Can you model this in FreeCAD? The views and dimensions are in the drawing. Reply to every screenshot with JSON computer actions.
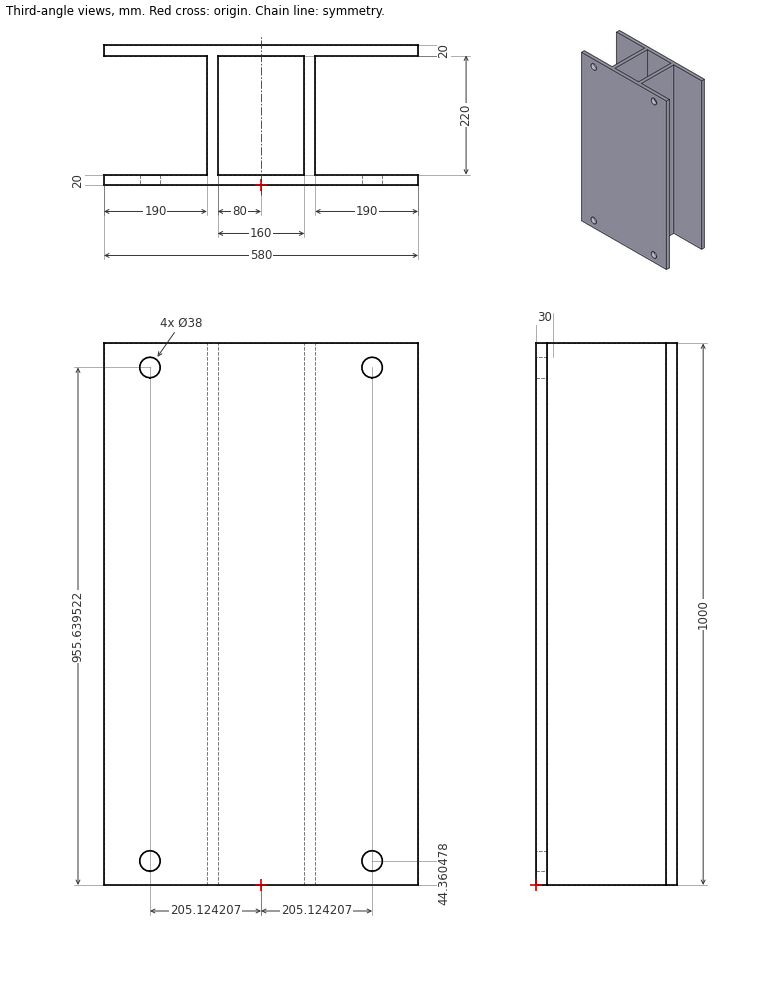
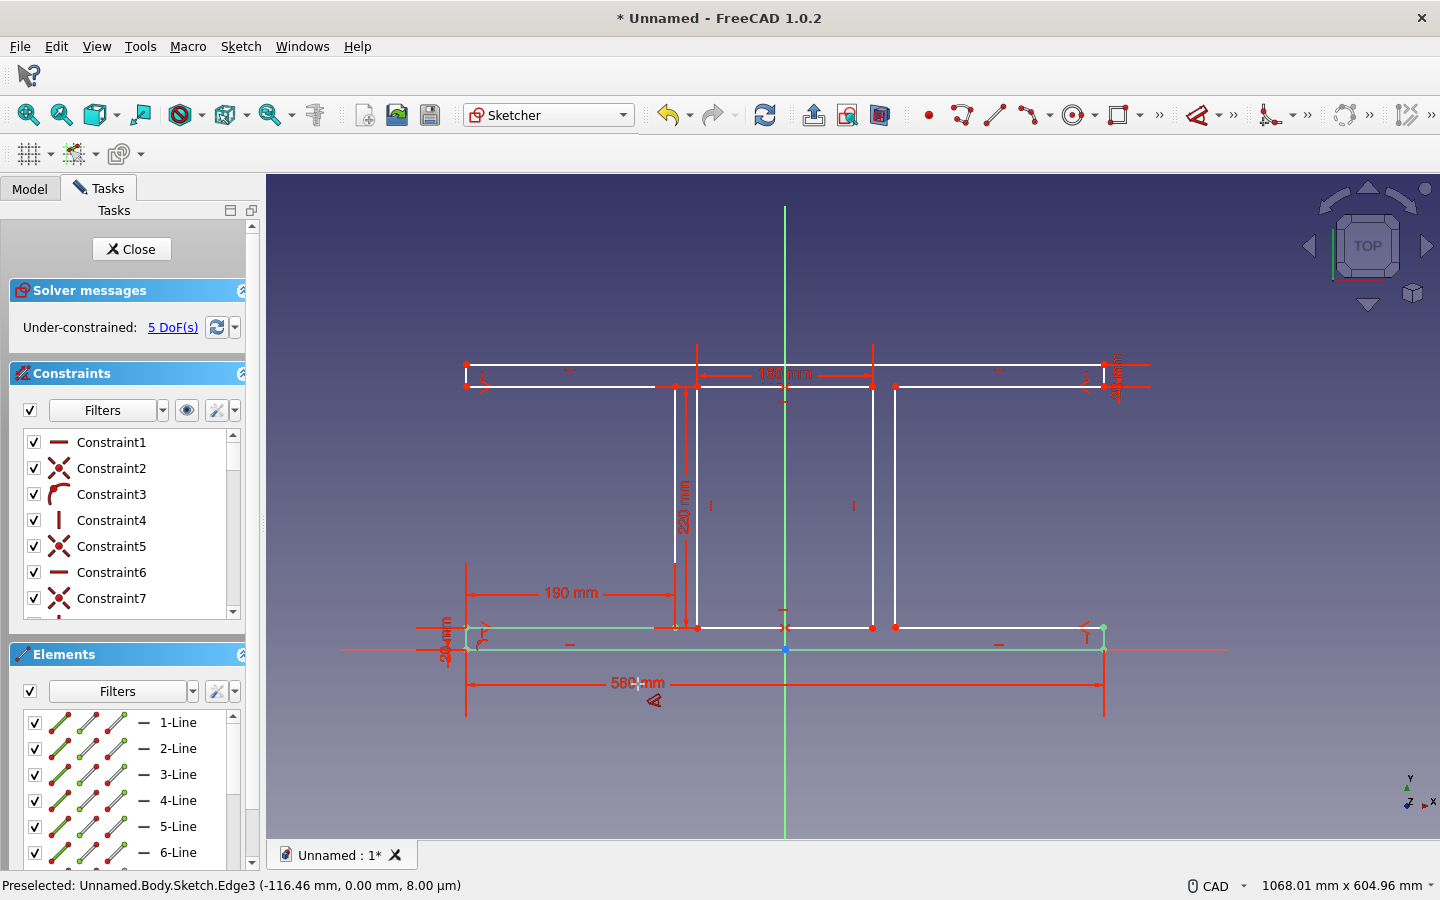
{"action": "left_click", "coordinate": [1041, 628]}
{"action": "left_click", "coordinate": [999, 594]}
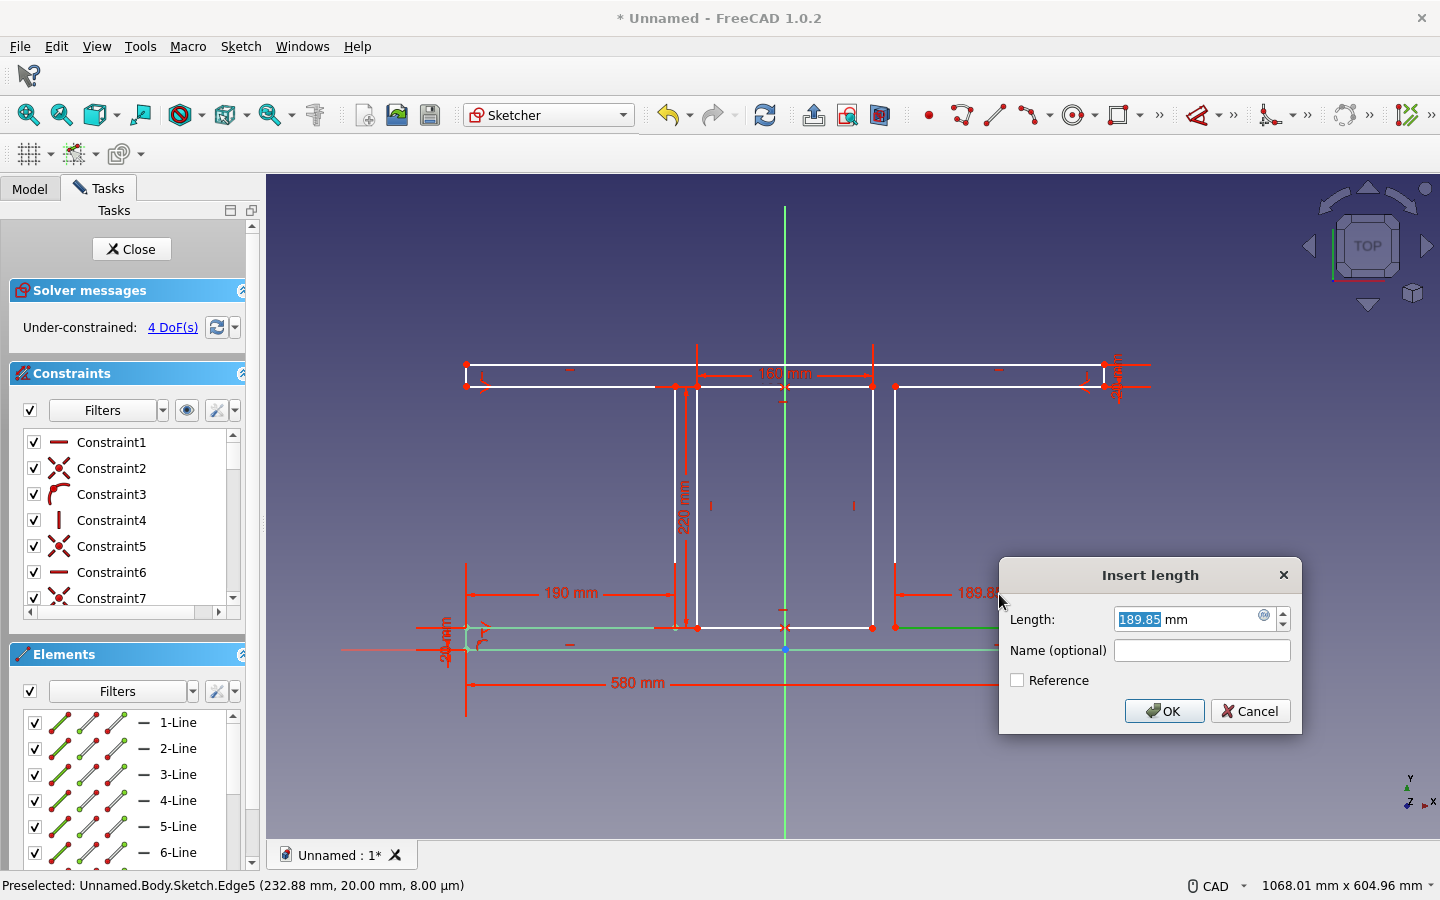
{"action": "type", "text": "190"}
{"action": "key", "text": "Return"}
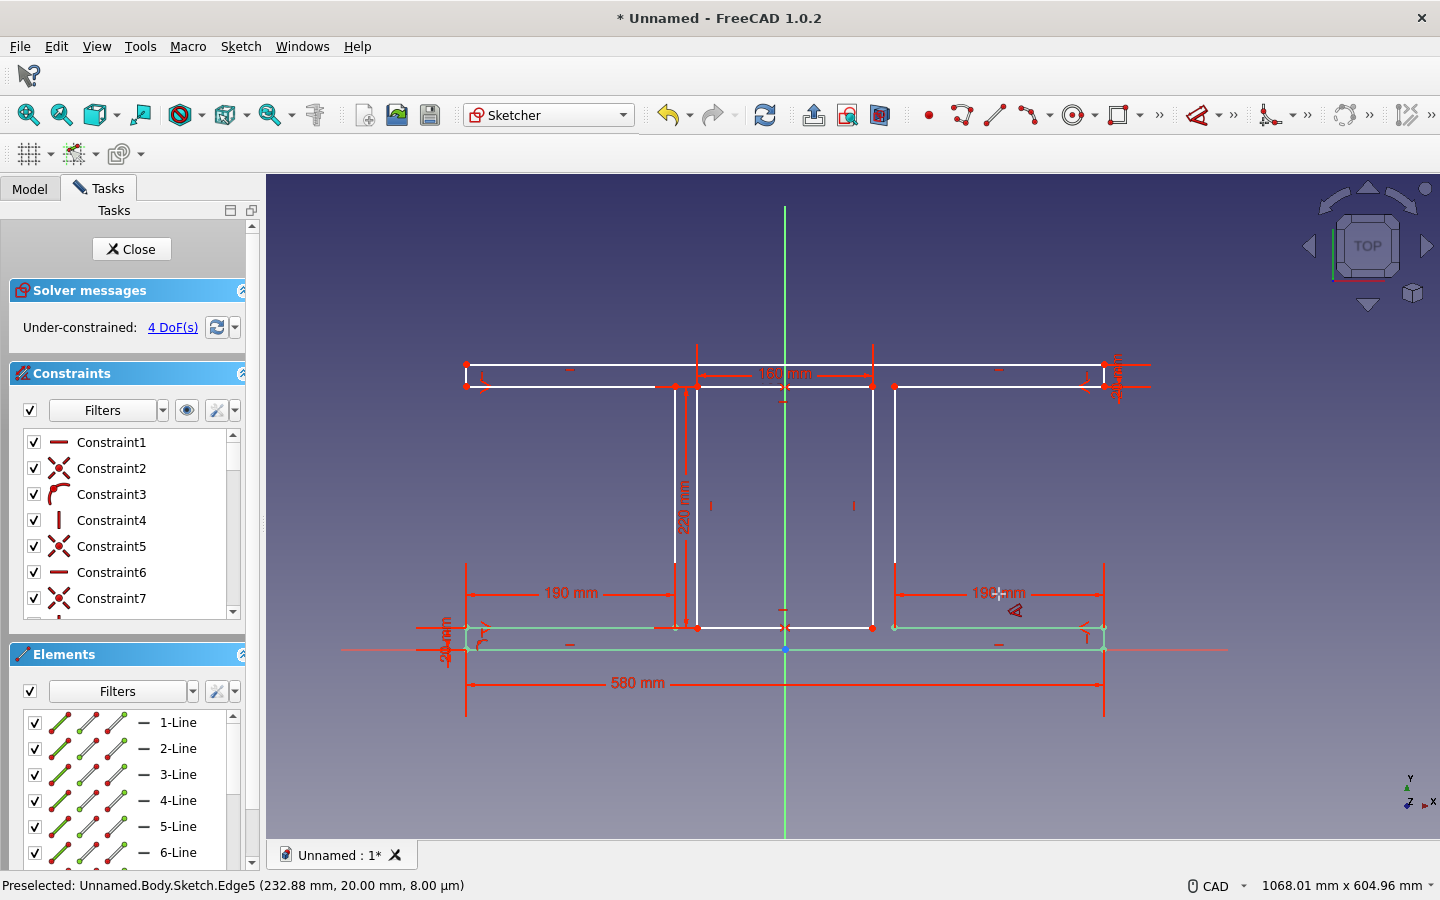
{"action": "left_click", "coordinate": [895, 555]}
{"action": "left_click", "coordinate": [929, 507]}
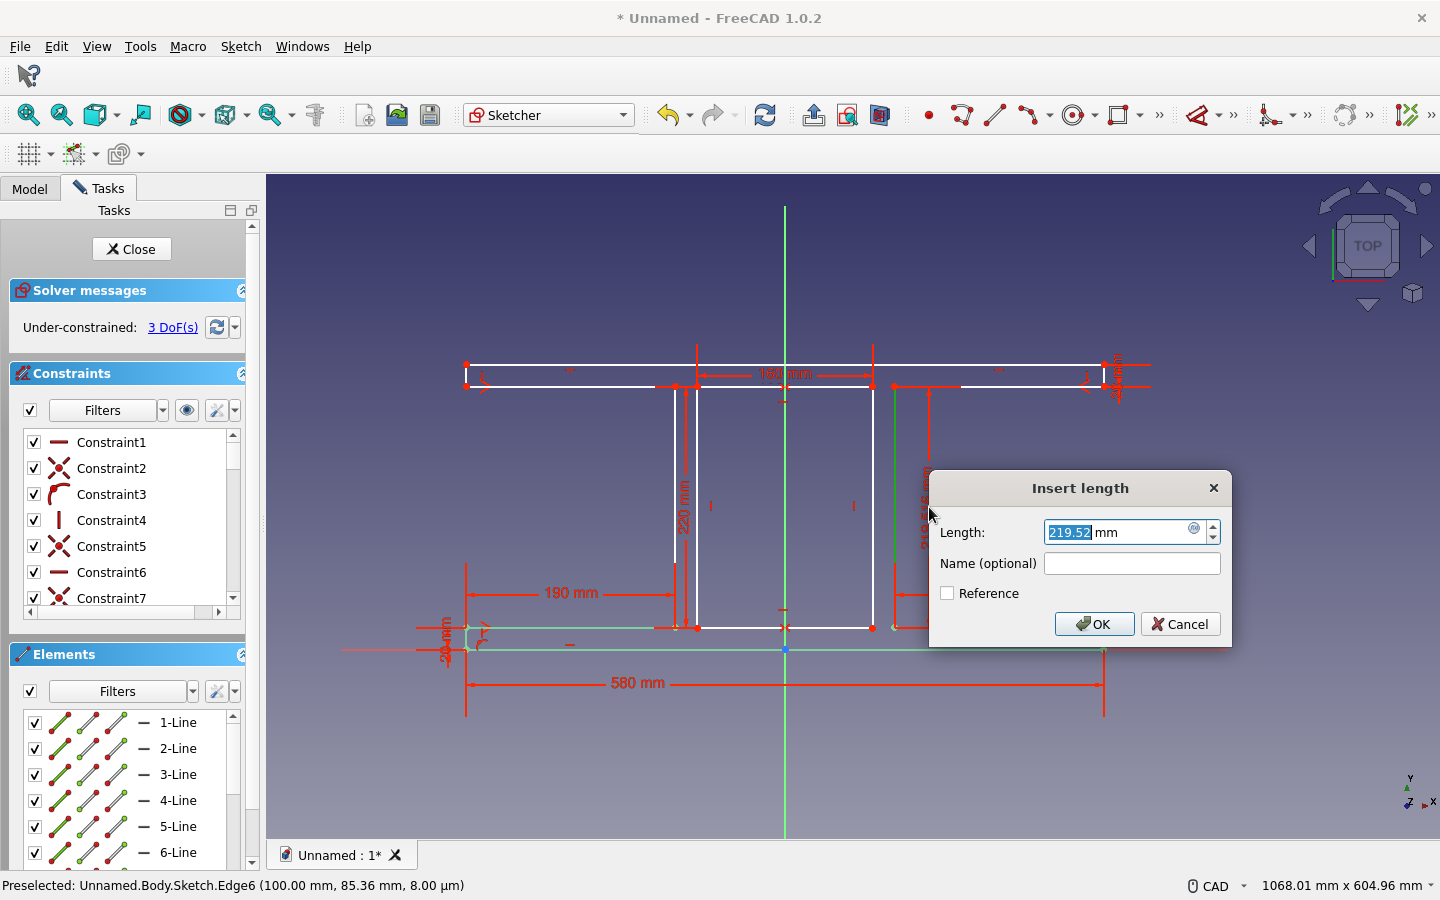
{"action": "type", "text": "220"}
{"action": "key", "text": "Return"}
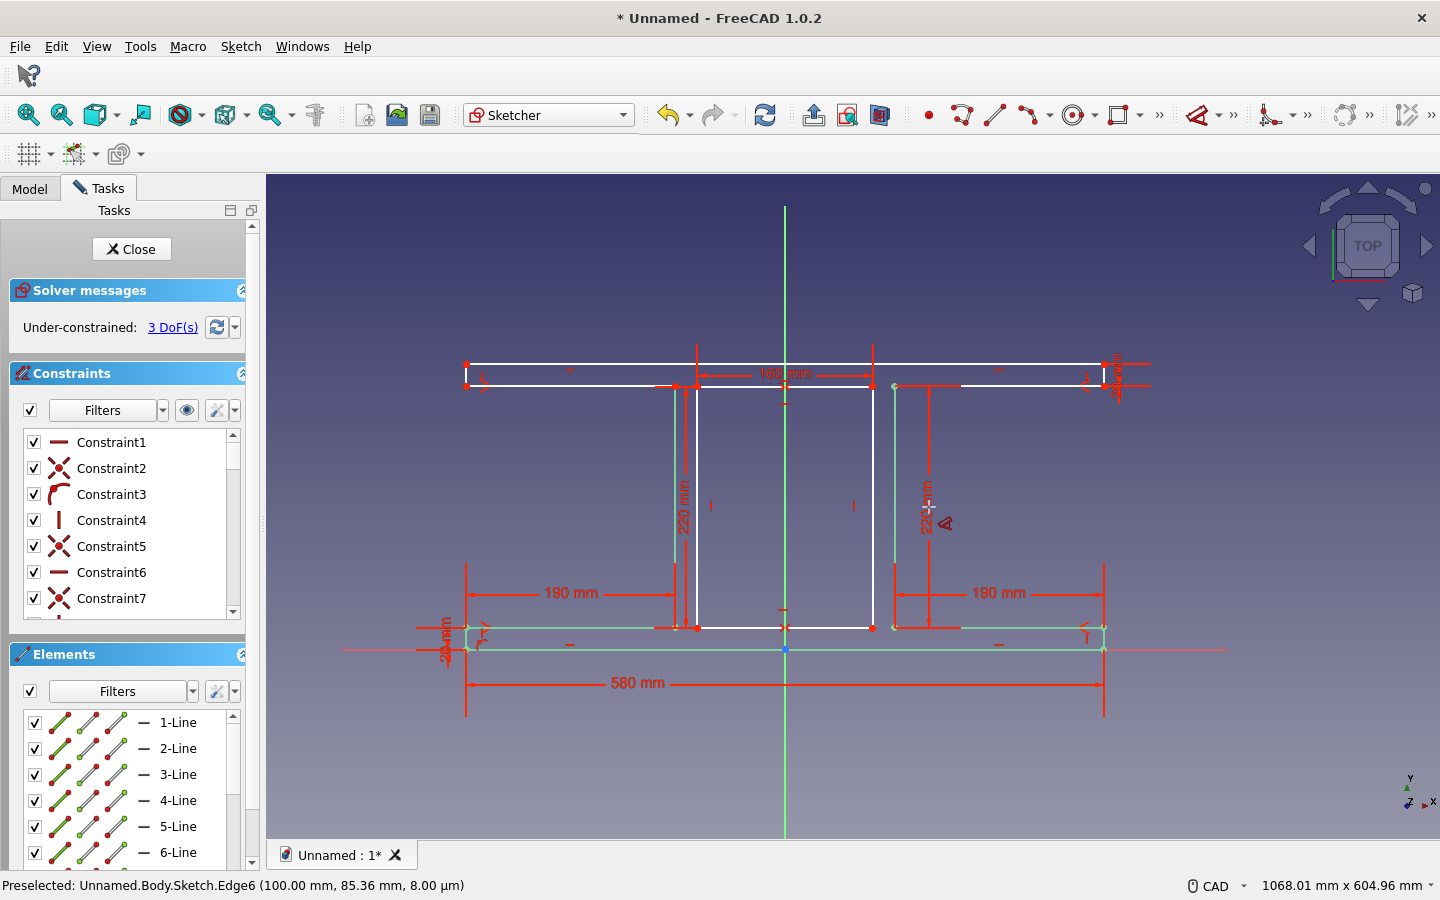
{"action": "left_click", "coordinate": [958, 386]}
{"action": "left_click", "coordinate": [999, 420]}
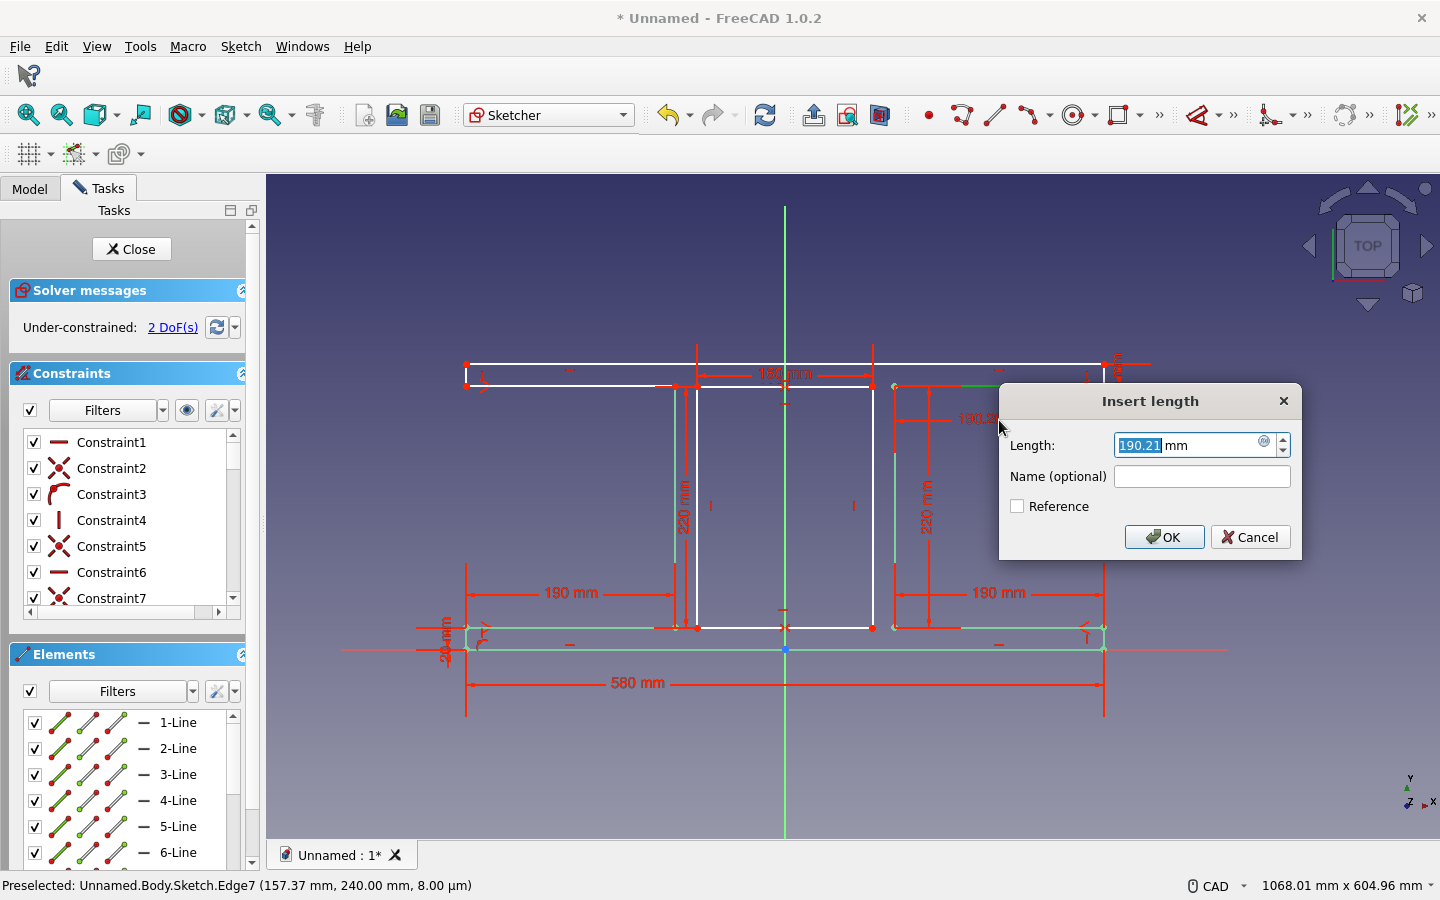
{"action": "type", "text": "190"}
{"action": "key", "text": "Return"}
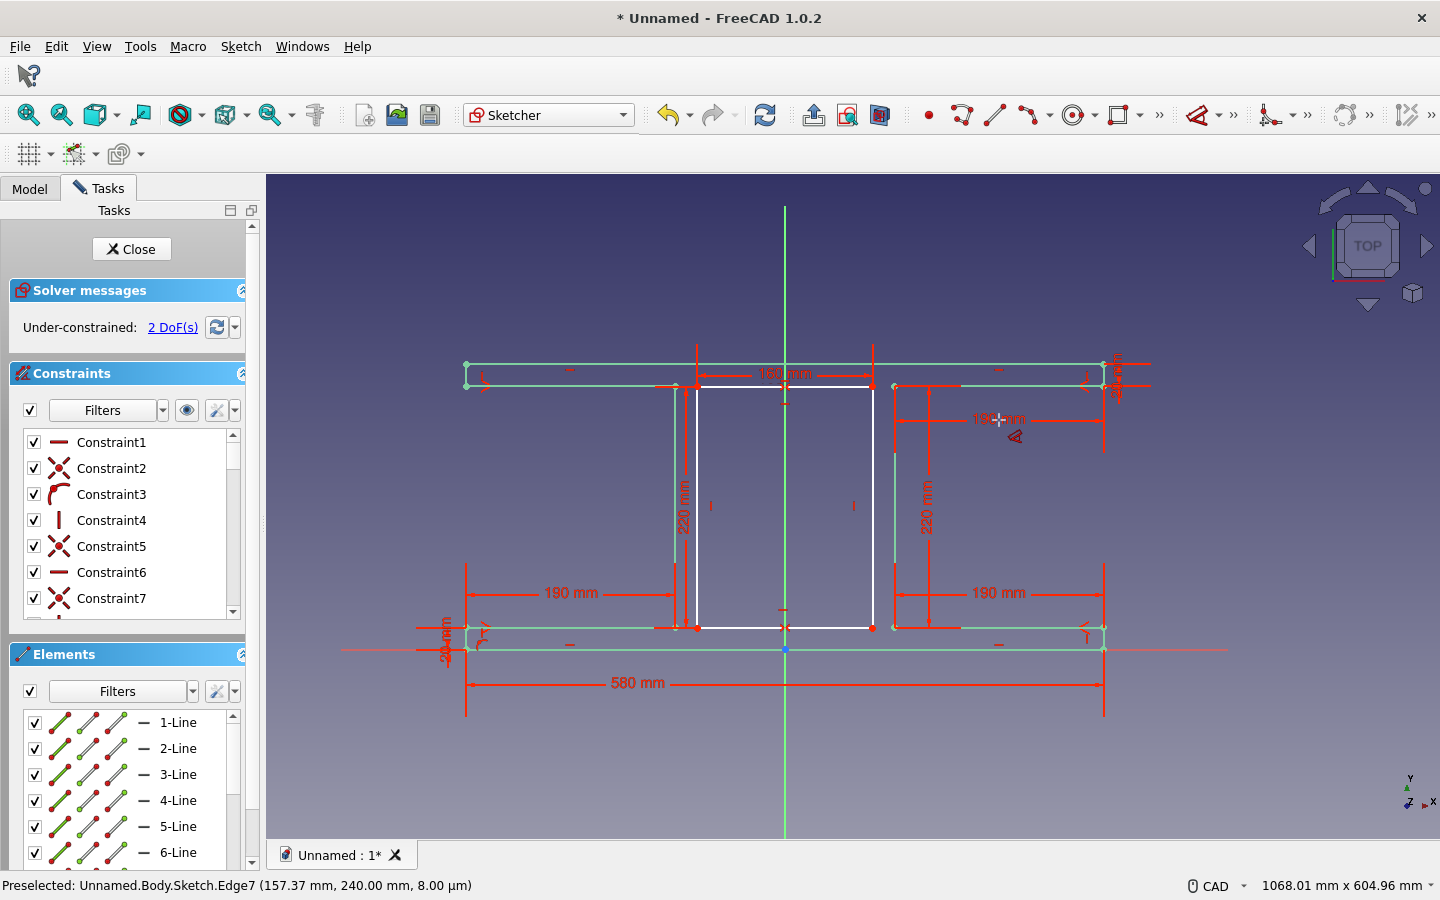
{"action": "left_click", "coordinate": [697, 387]}
{"action": "left_click", "coordinate": [741, 684]}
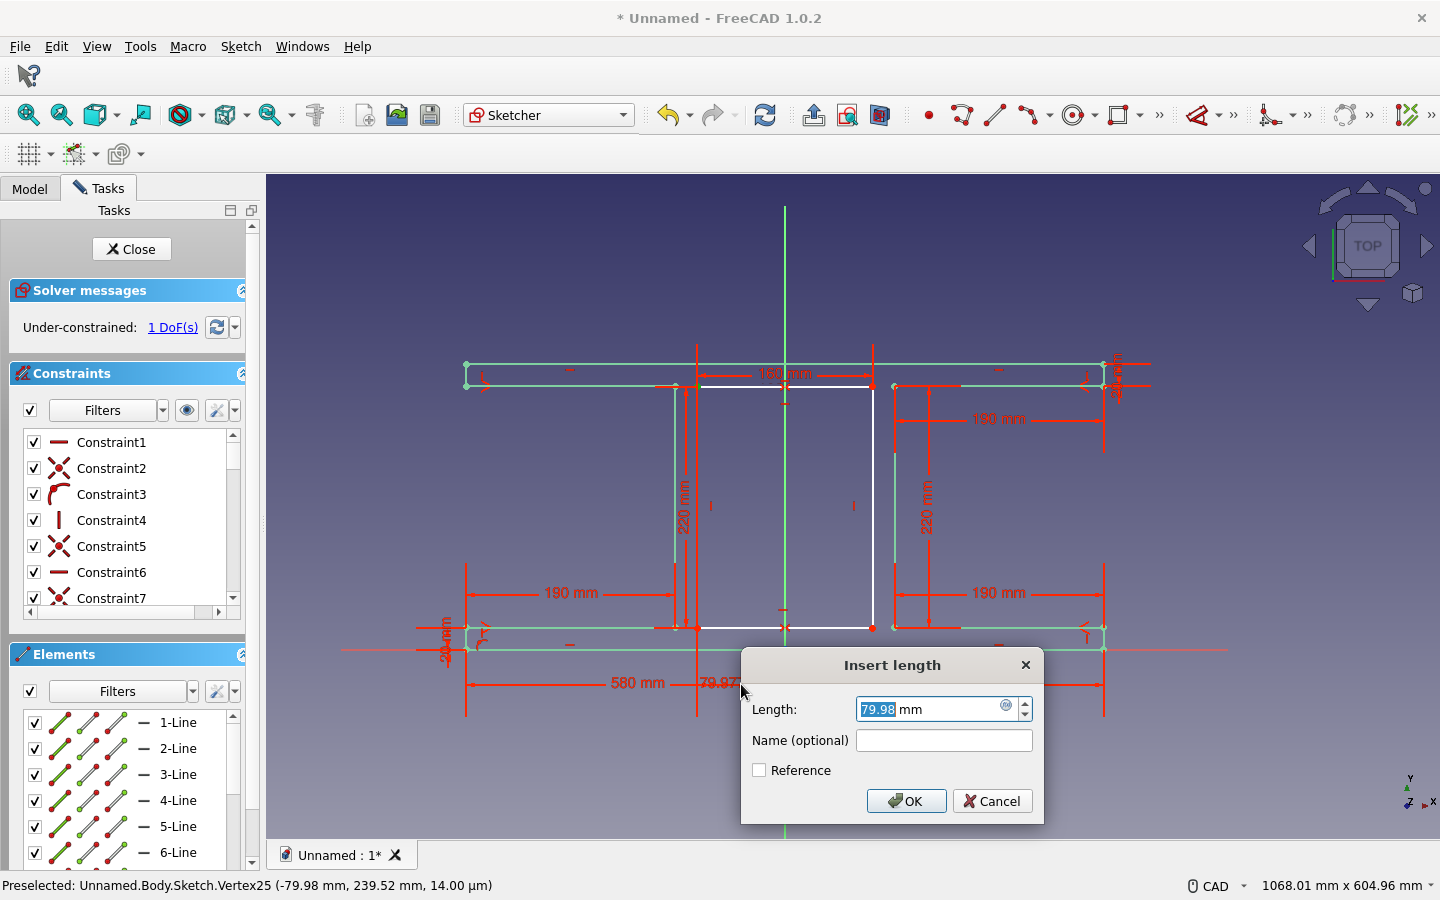
{"action": "type", "text": "80"}
{"action": "key", "text": "Return"}